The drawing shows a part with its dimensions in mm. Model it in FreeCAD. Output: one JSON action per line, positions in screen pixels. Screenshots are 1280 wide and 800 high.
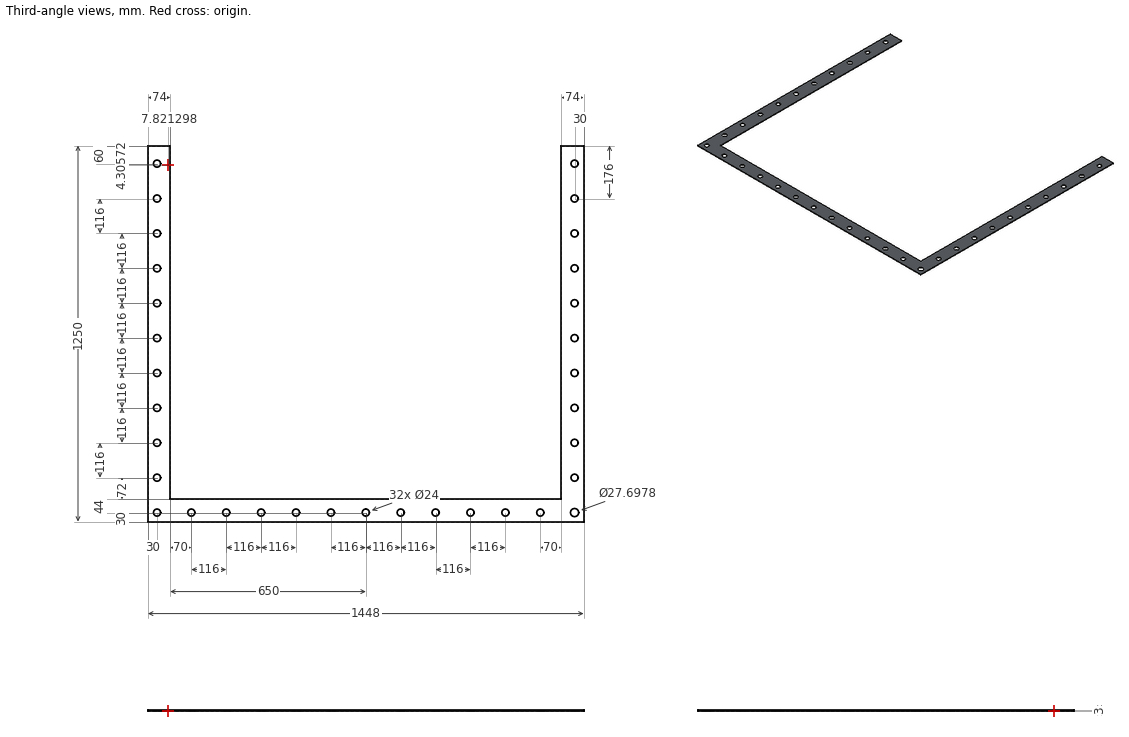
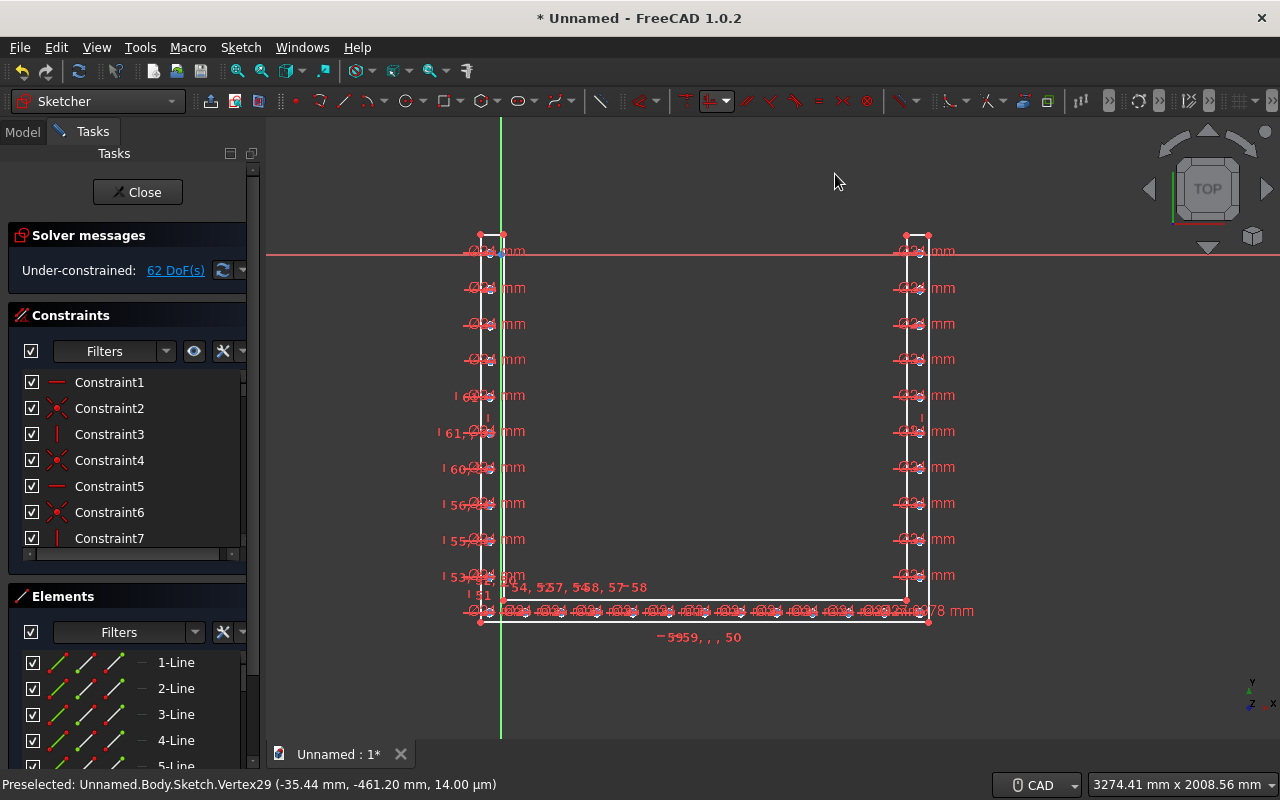
{"action": "left_click", "coordinate": [490, 397]}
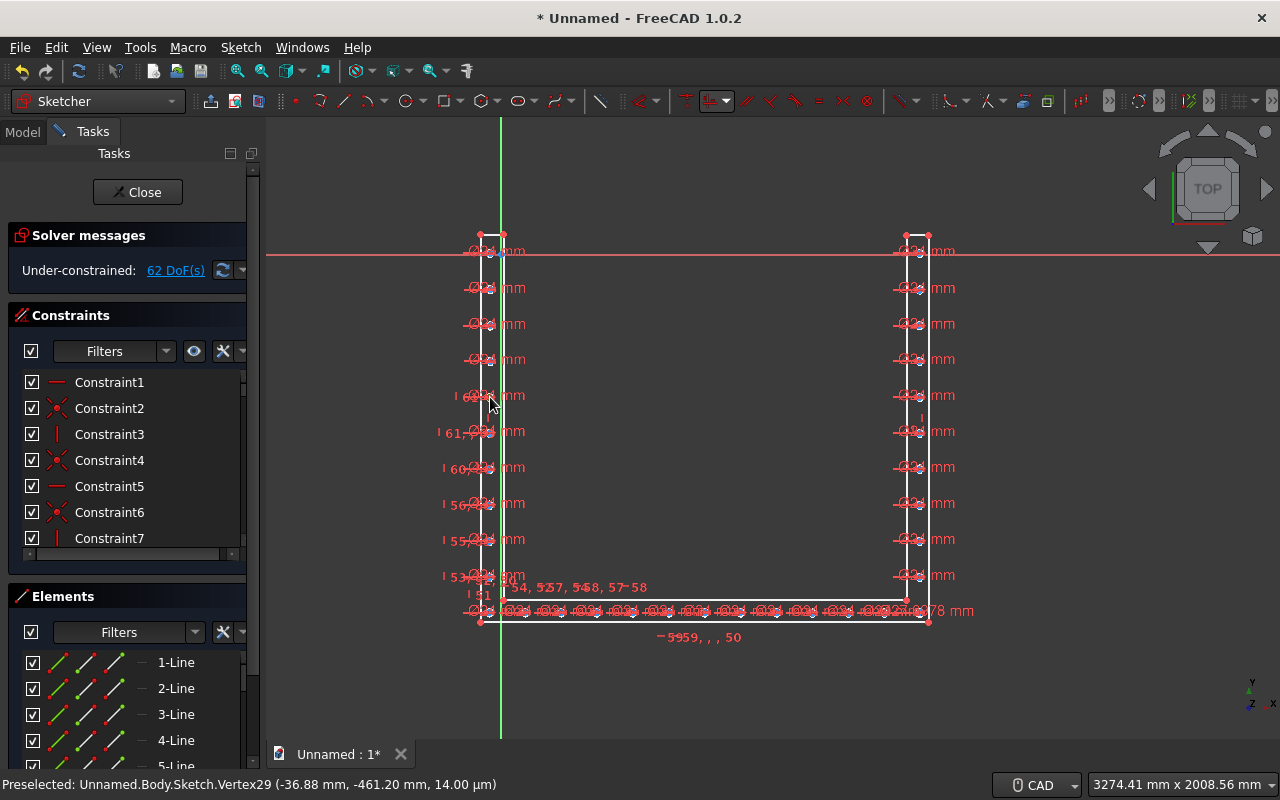
{"action": "left_click", "coordinate": [490, 361]}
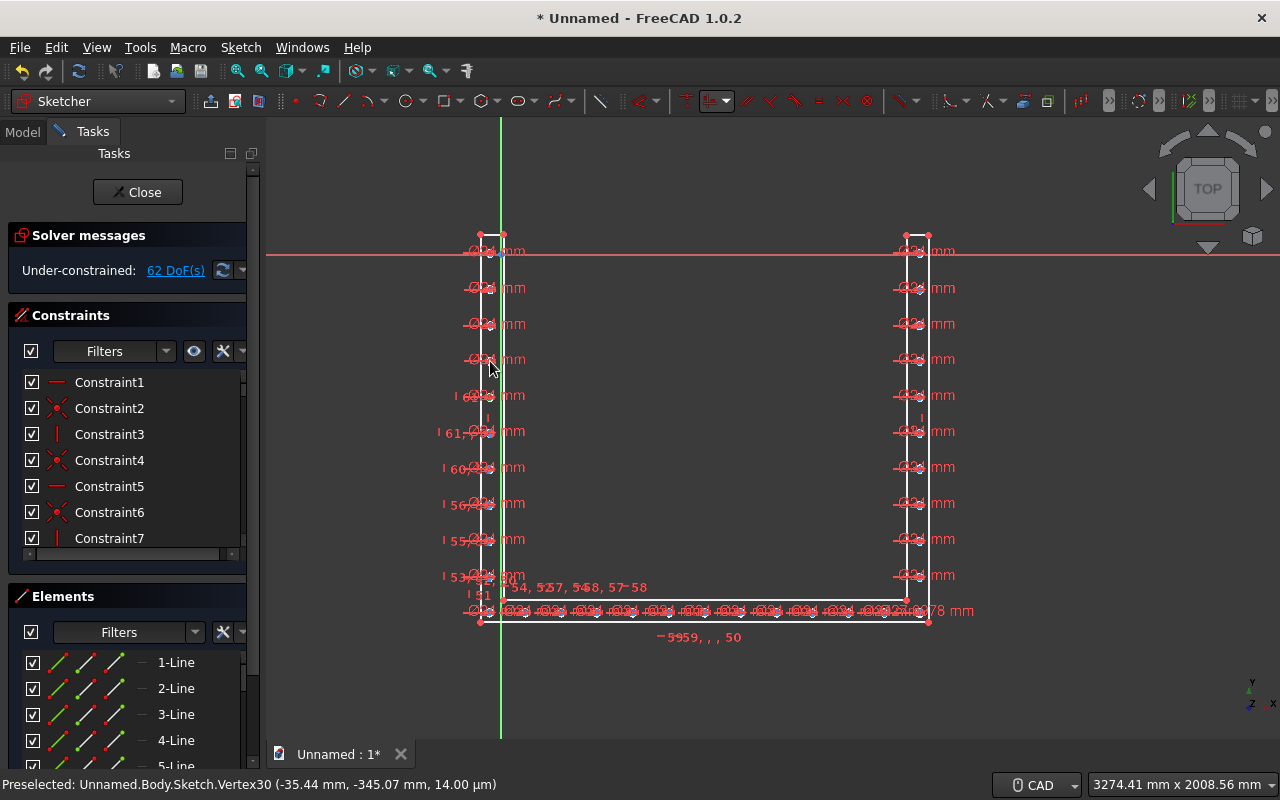
{"action": "key", "text": "v"}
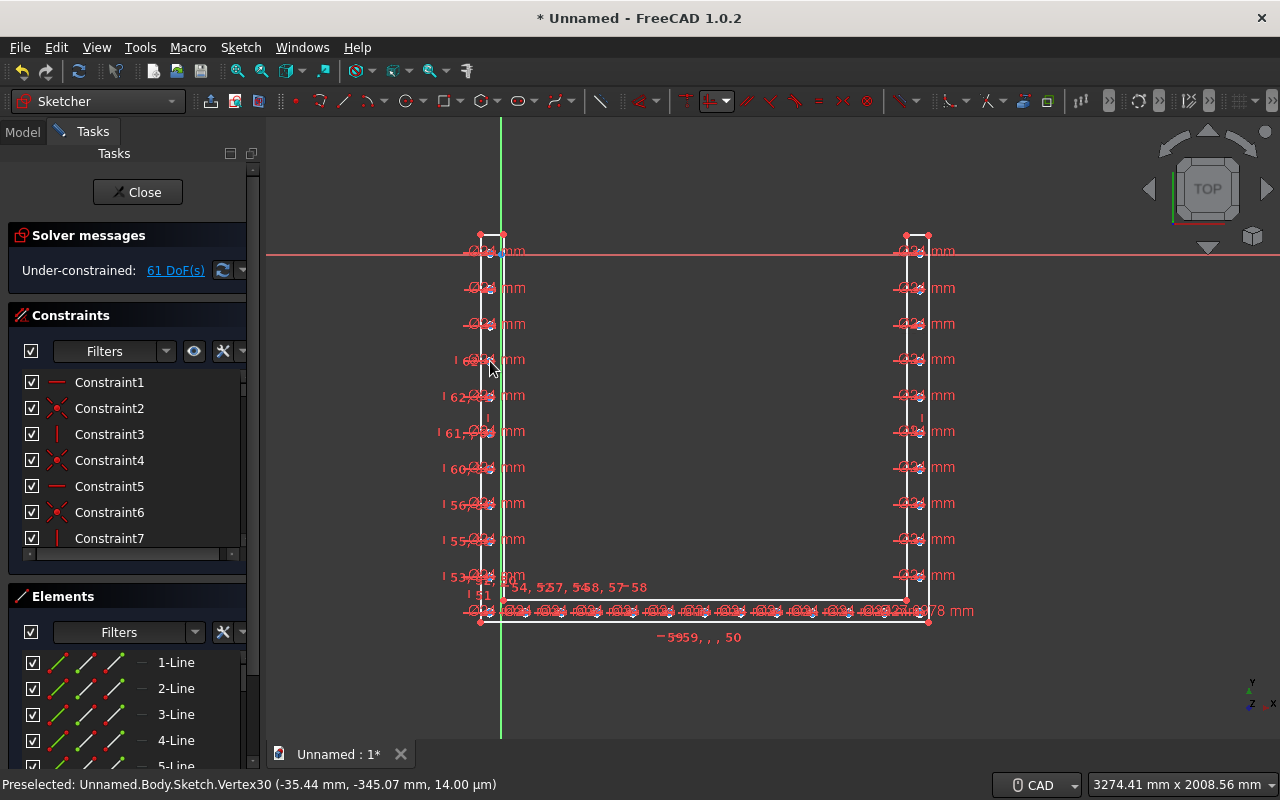
{"action": "left_click", "coordinate": [490, 361]}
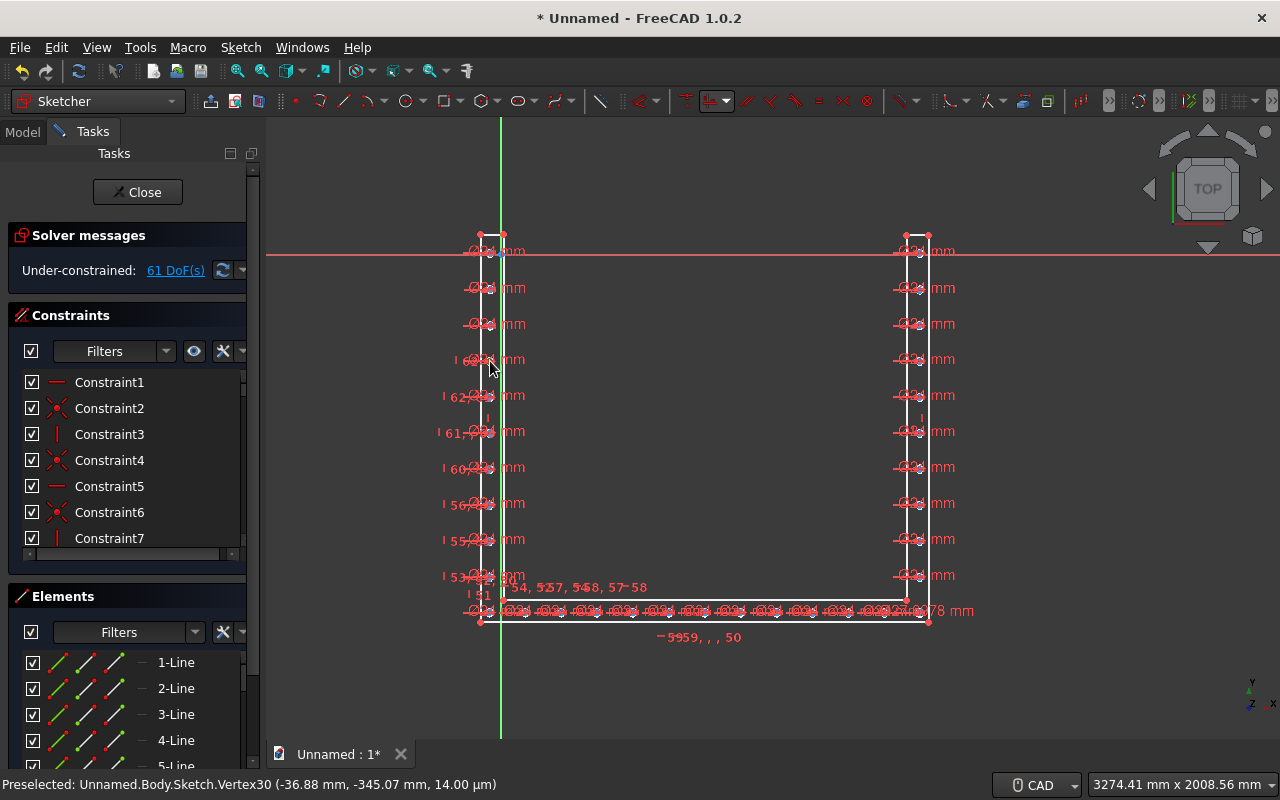
{"action": "left_click", "coordinate": [490, 326]}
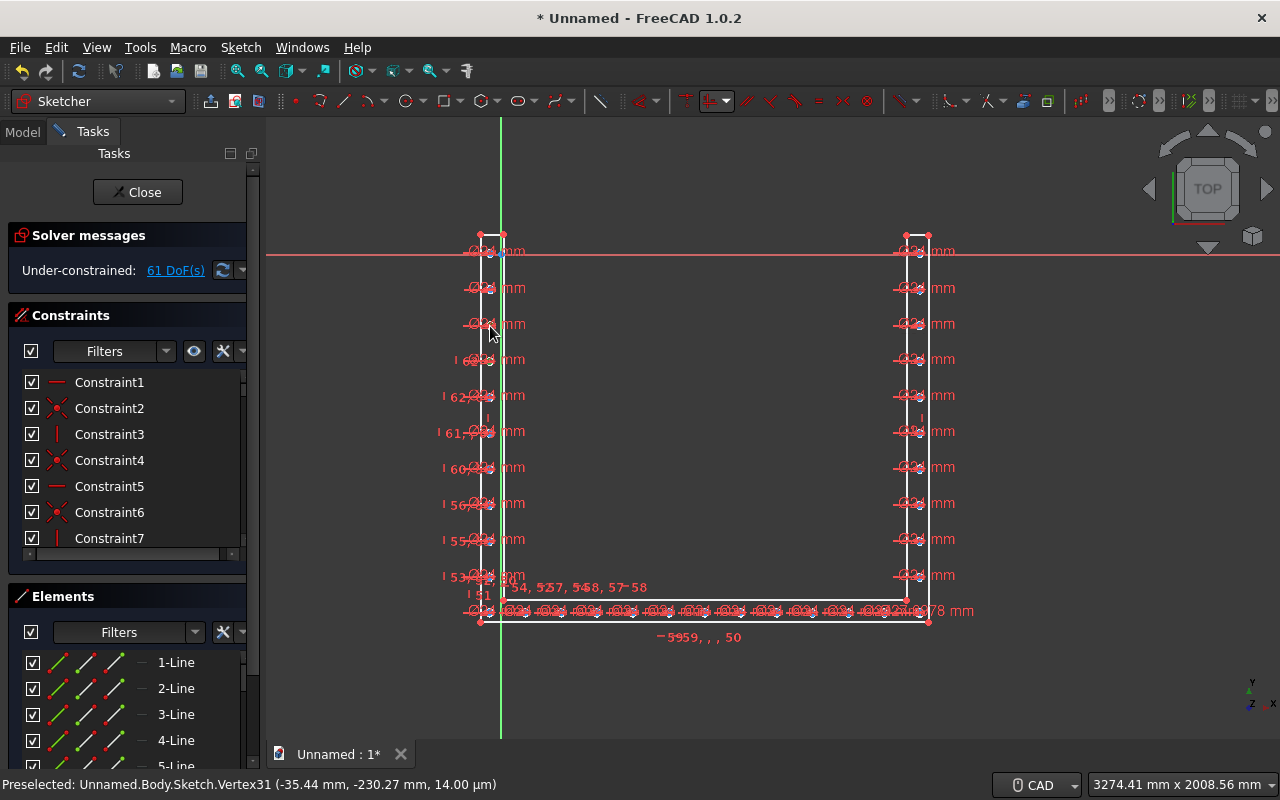
{"action": "left_click", "coordinate": [728, 102]}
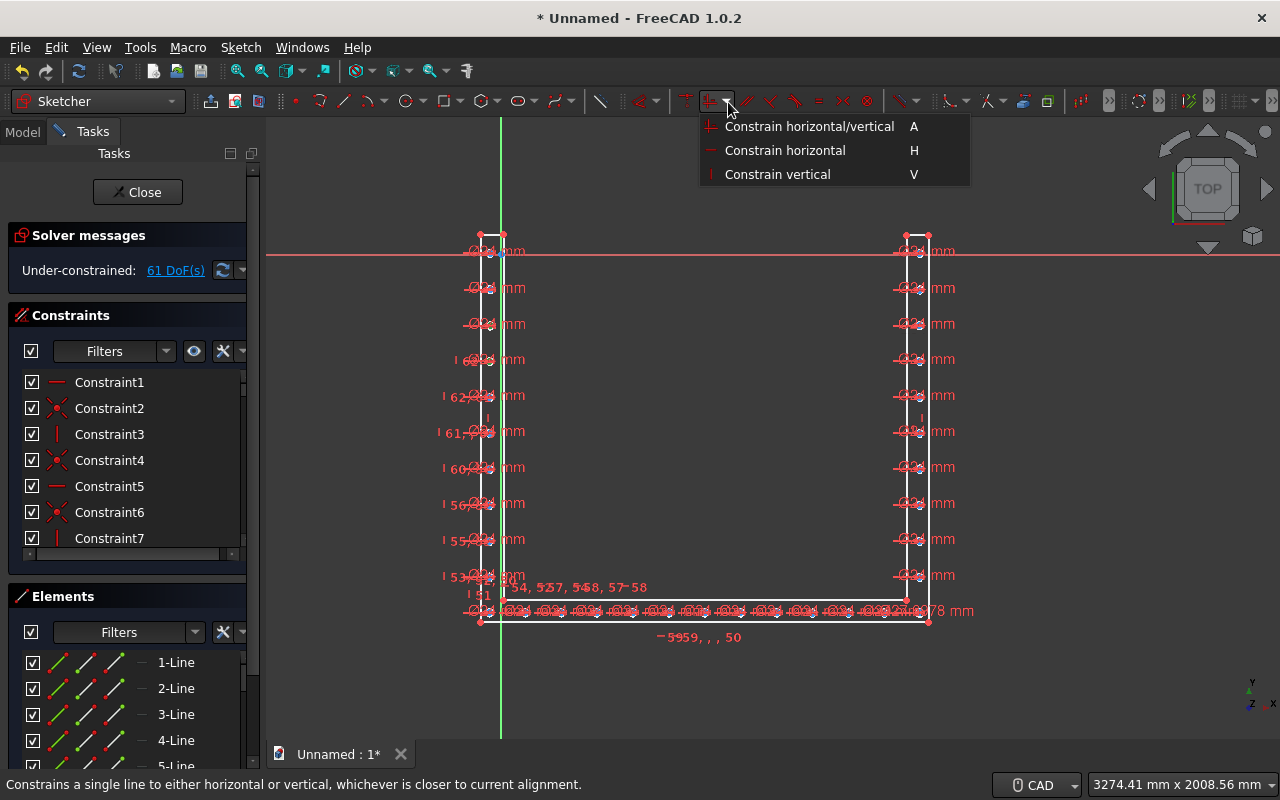
{"action": "left_click", "coordinate": [835, 174]}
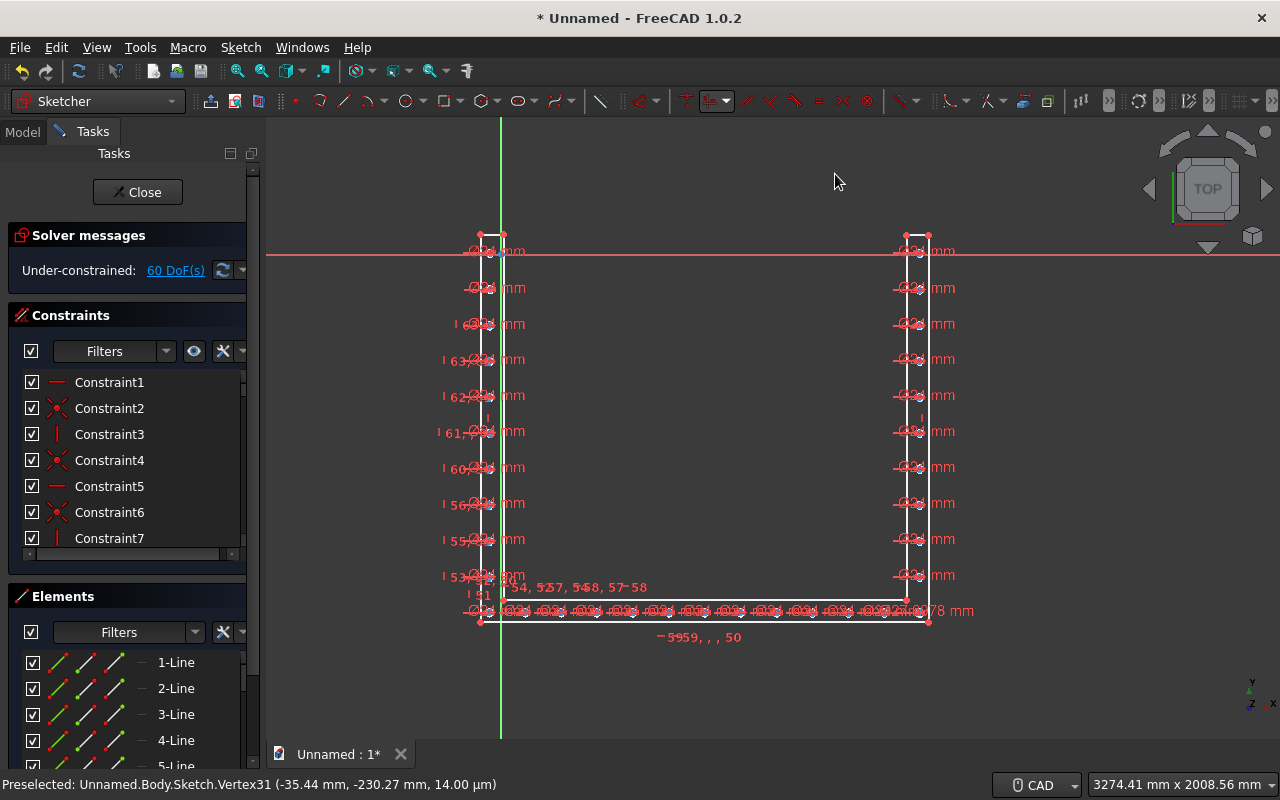
{"action": "left_click", "coordinate": [490, 326]}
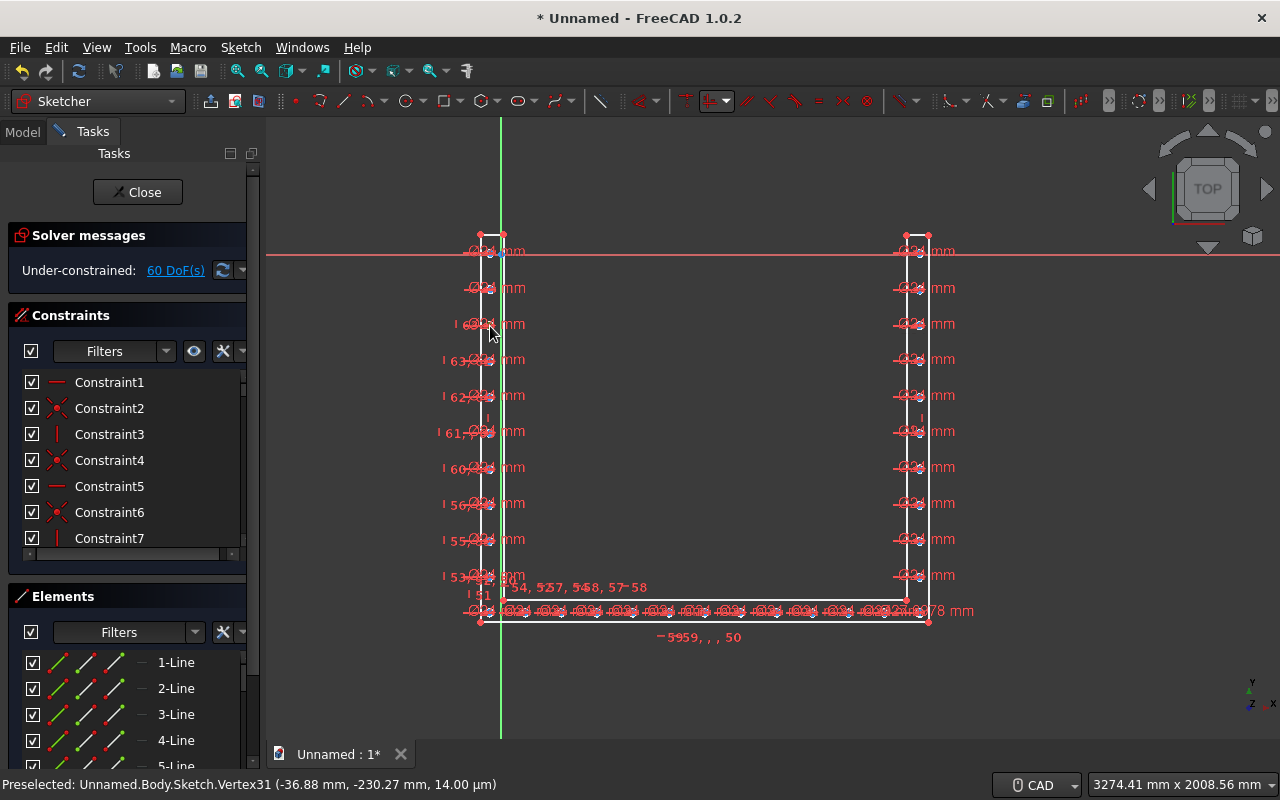
{"action": "left_click", "coordinate": [490, 290]}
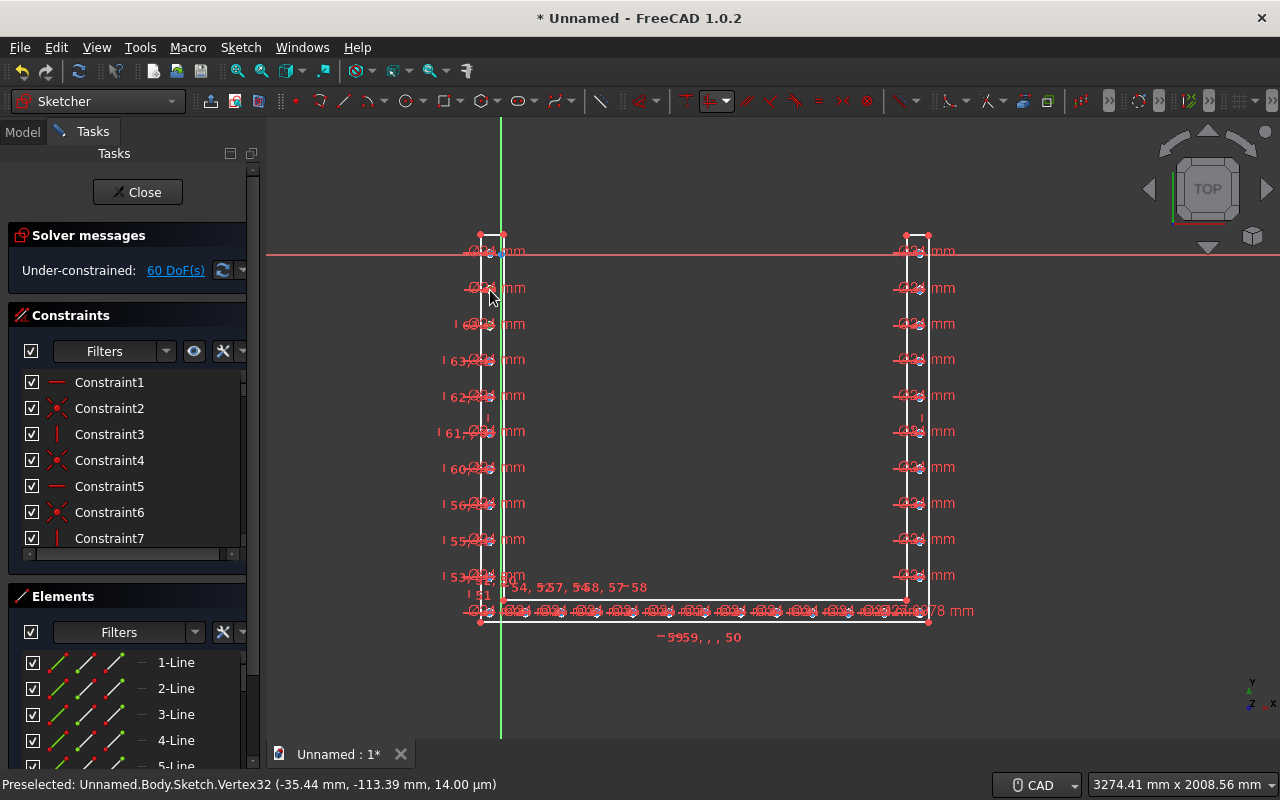
{"action": "left_click", "coordinate": [728, 102]}